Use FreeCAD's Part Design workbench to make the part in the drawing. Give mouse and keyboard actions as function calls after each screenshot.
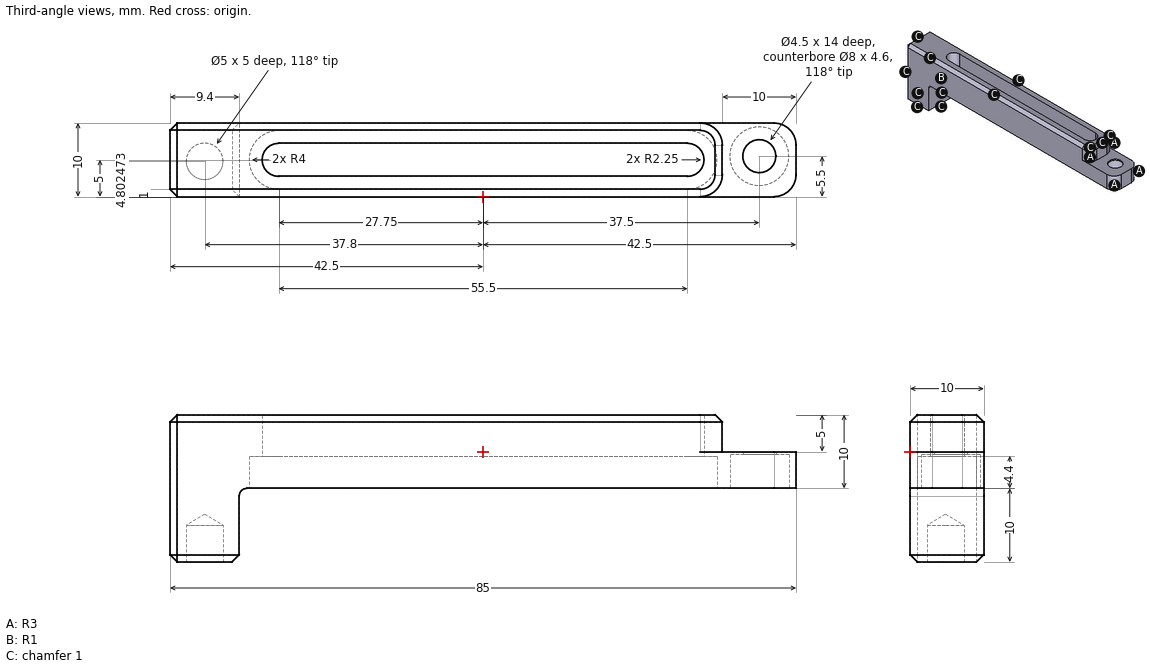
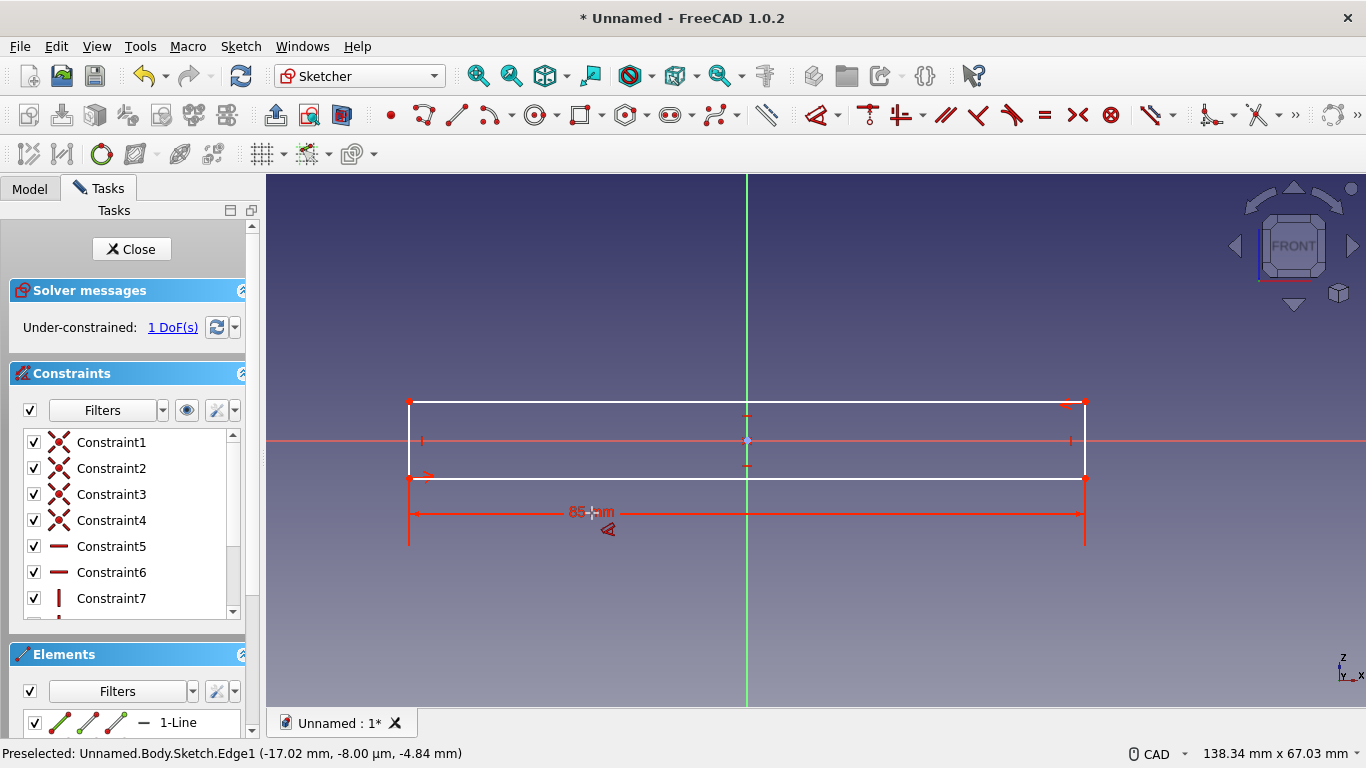
click(1085, 456)
click(1119, 423)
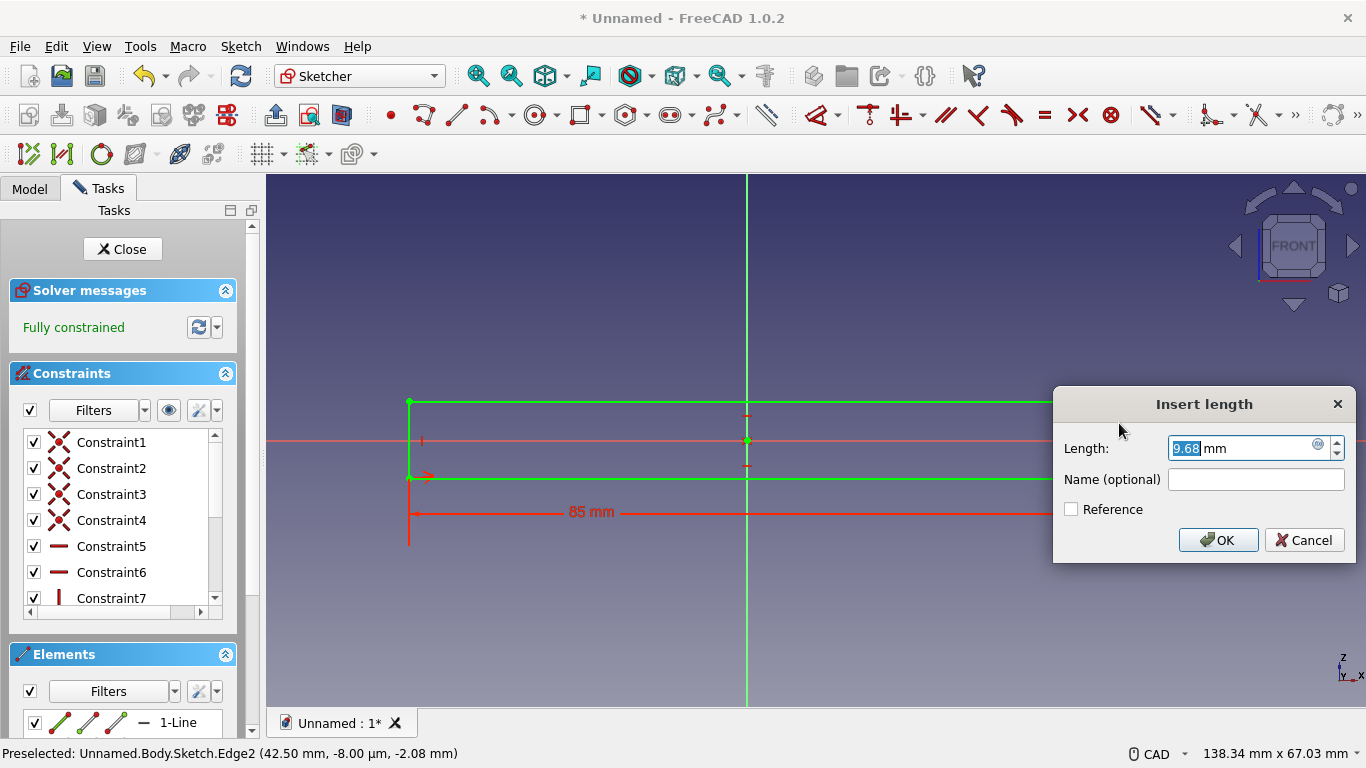
text(10)
key(Return)
key(Escape)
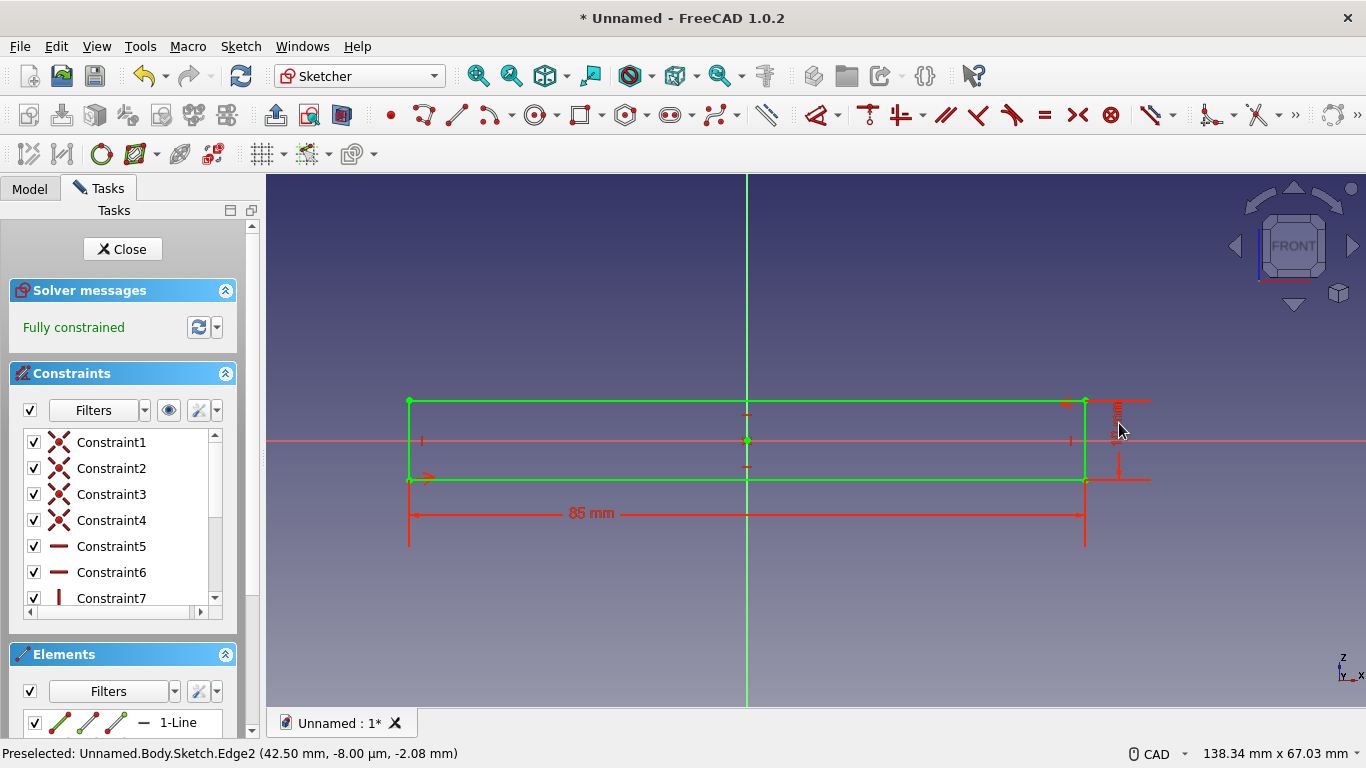
click(123, 249)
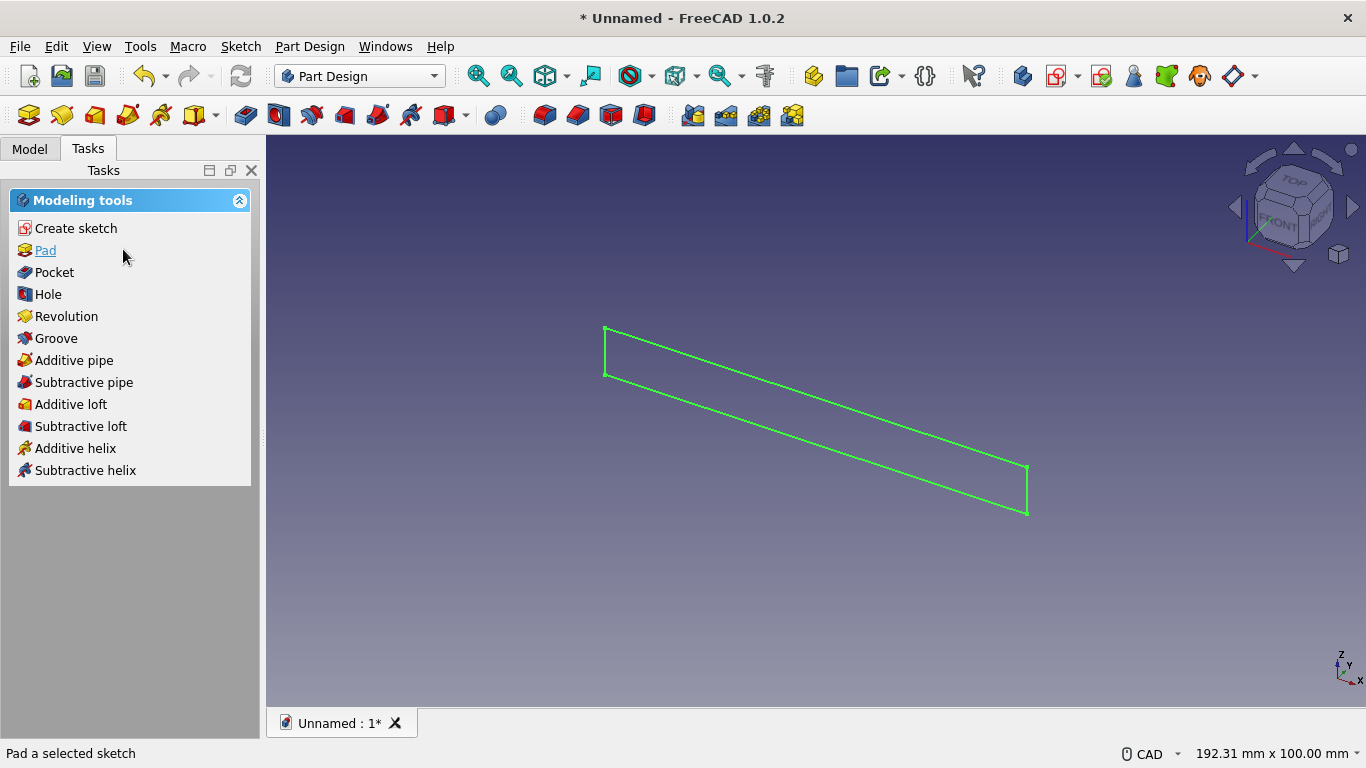
click(29, 116)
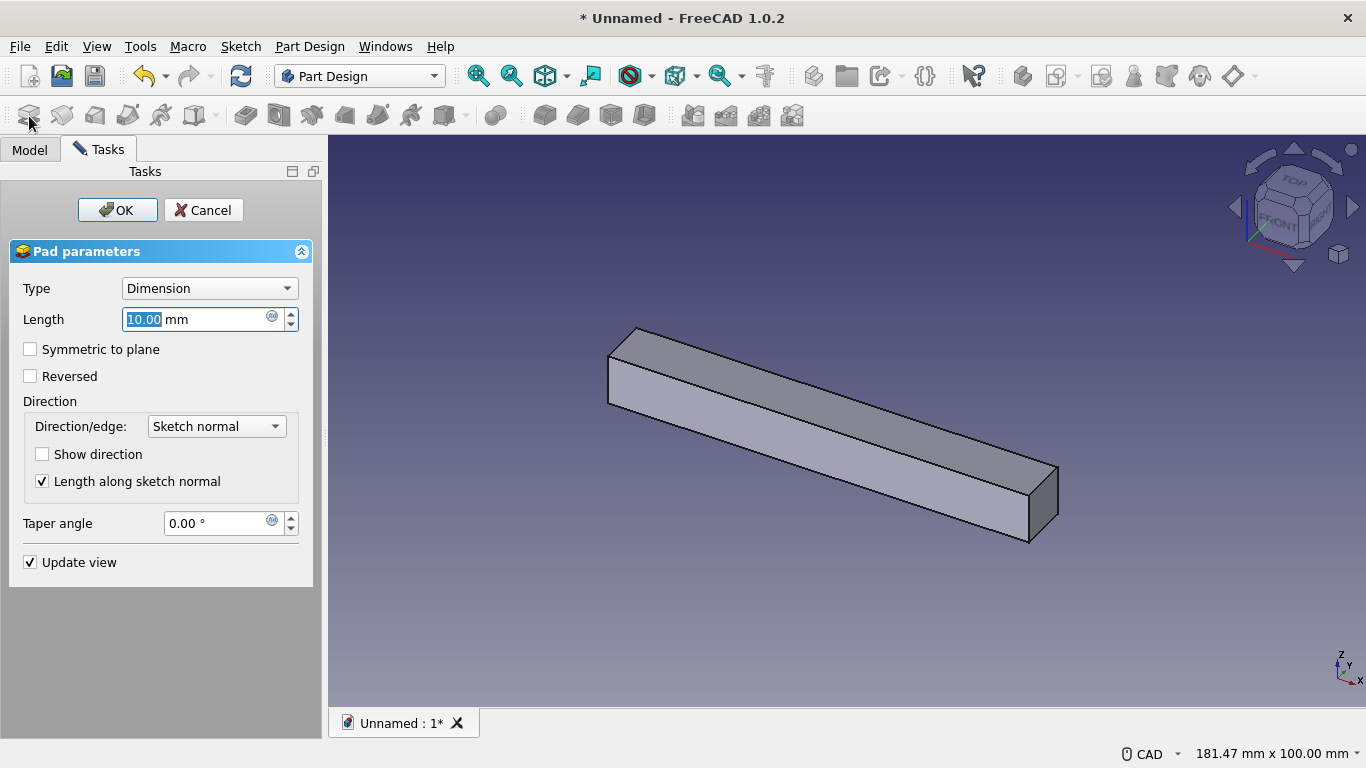
text(10)
key(Tab)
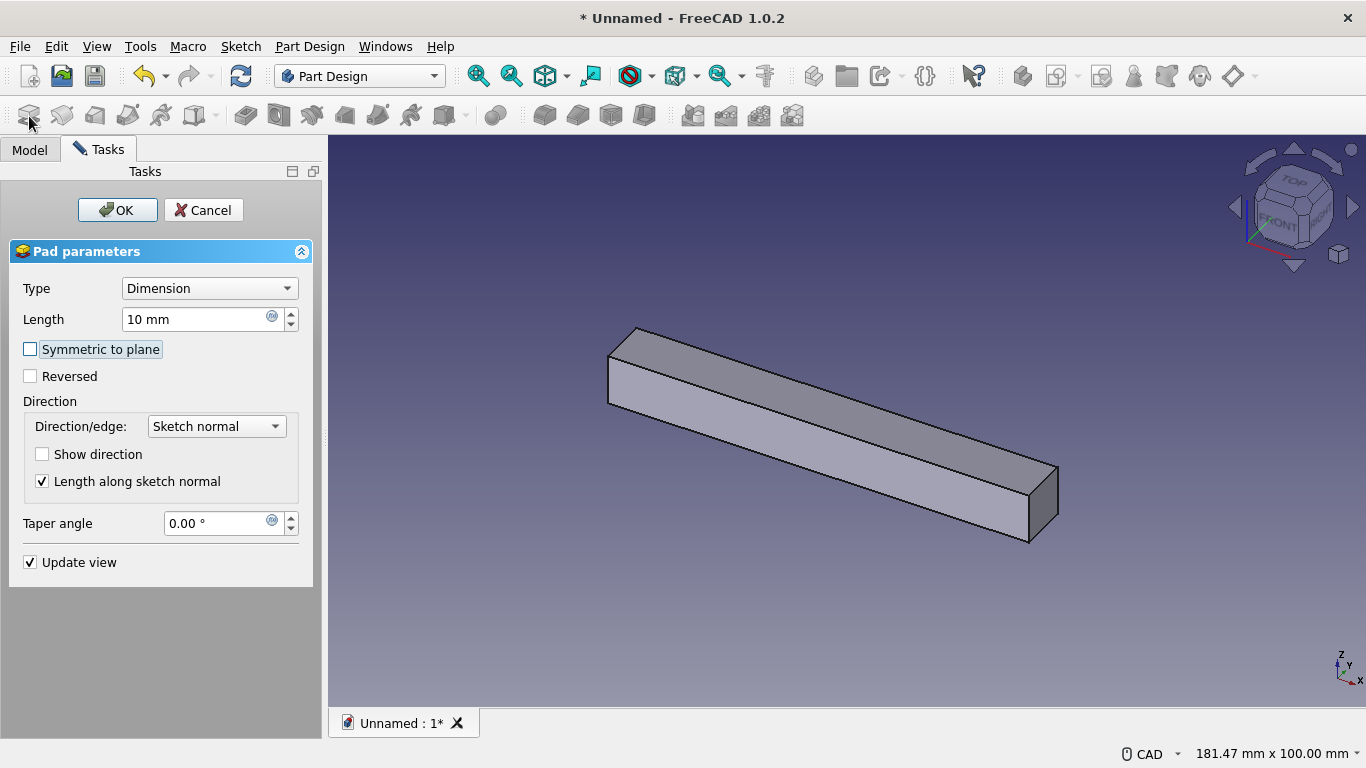
click(31, 376)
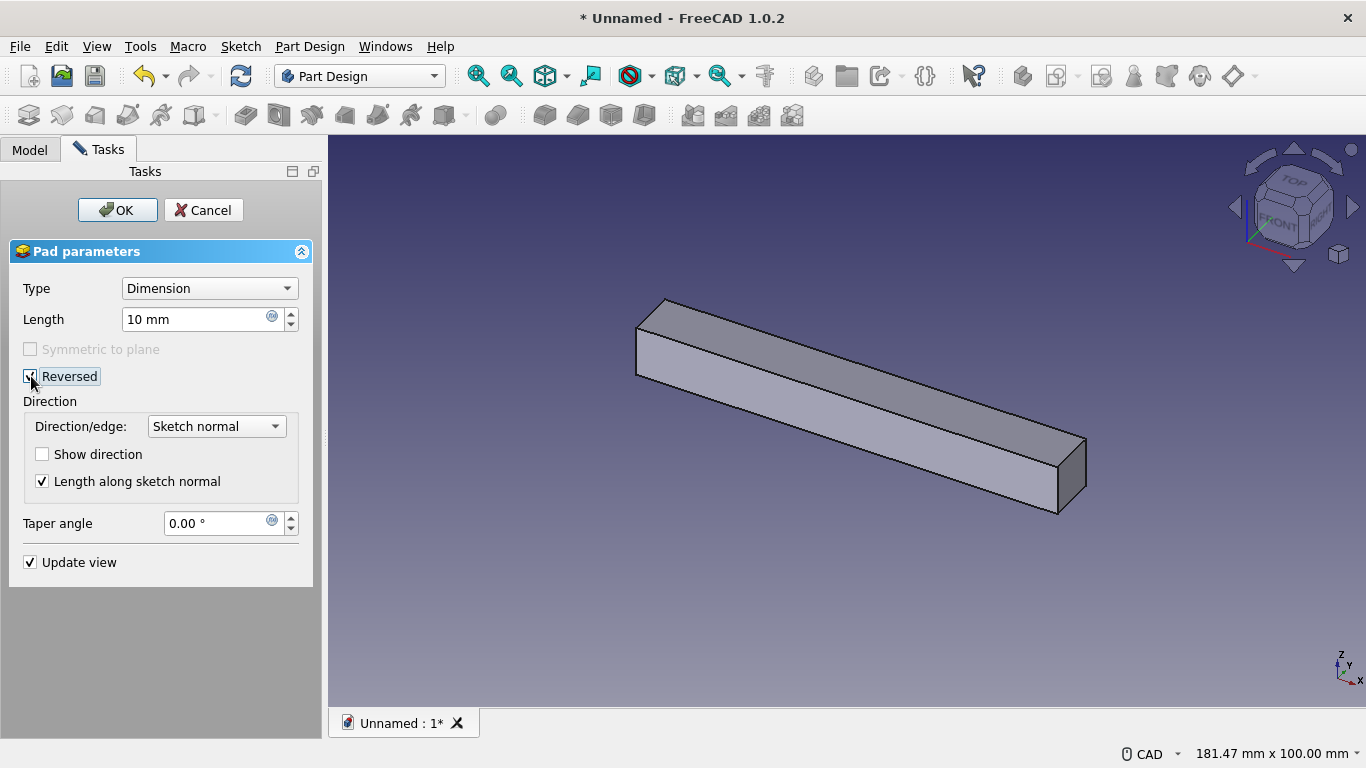
click(118, 210)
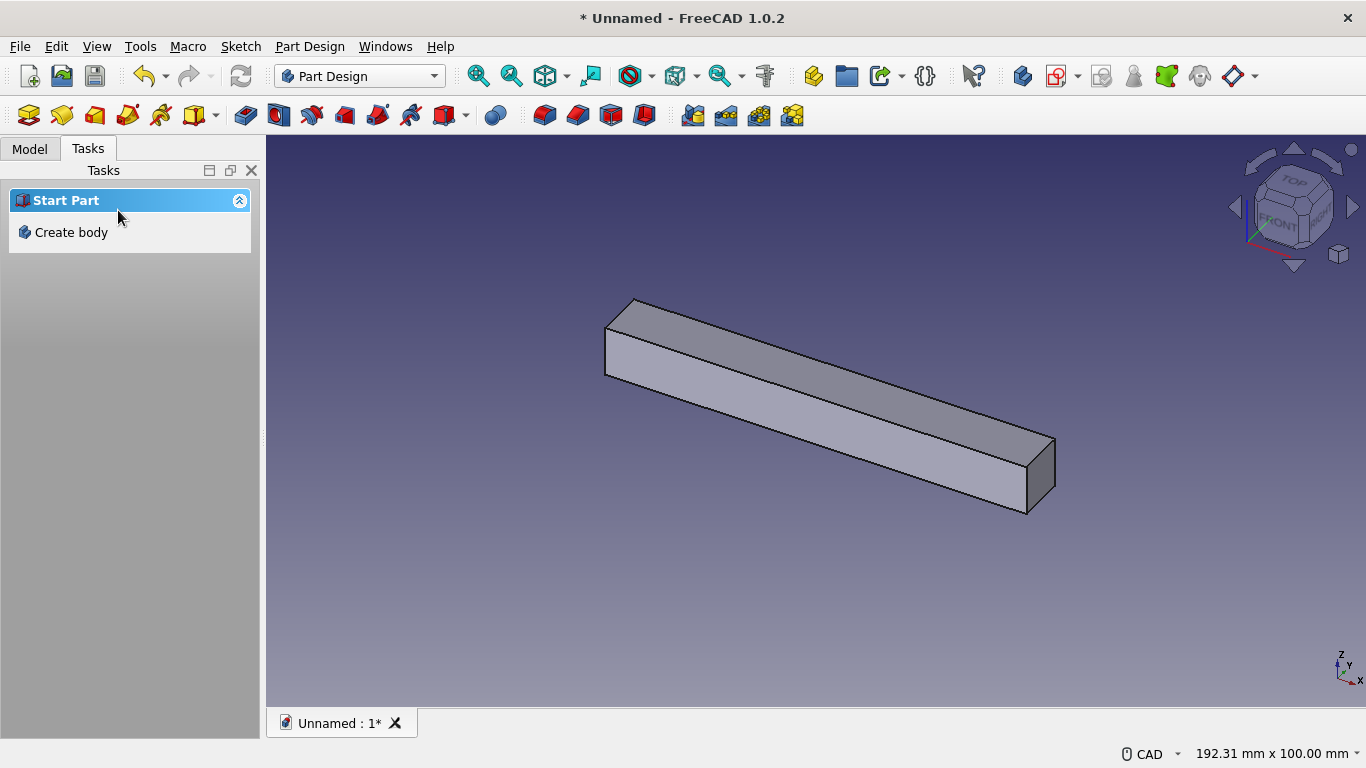
key(v)
key(f)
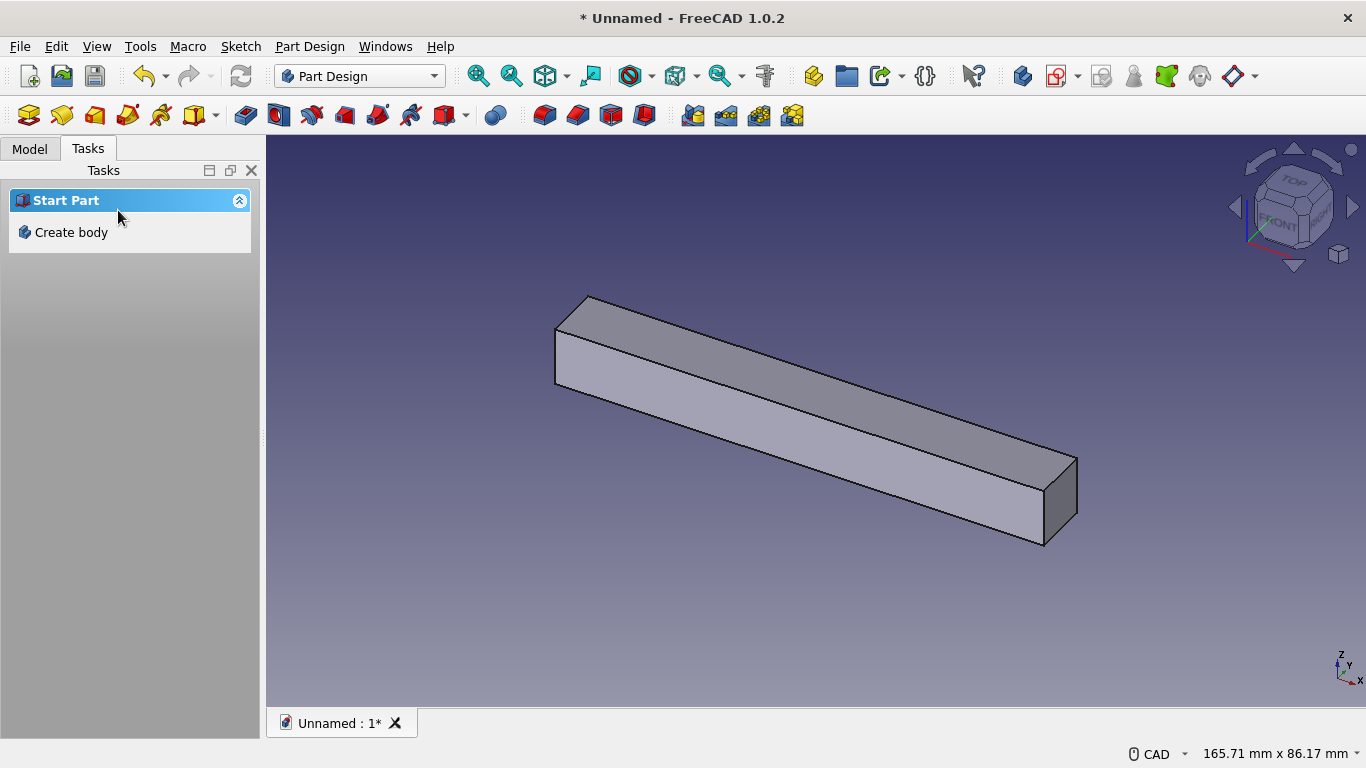
key(5)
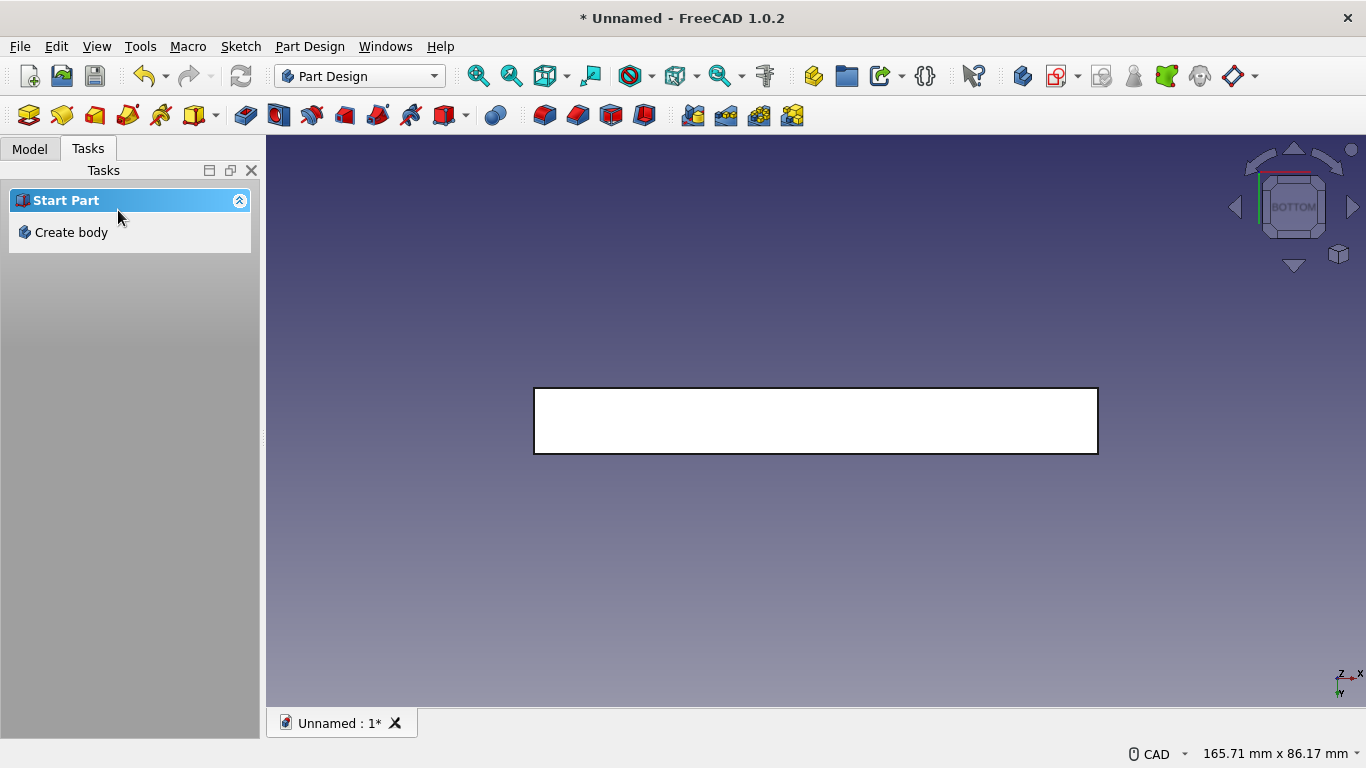
click(1058, 420)